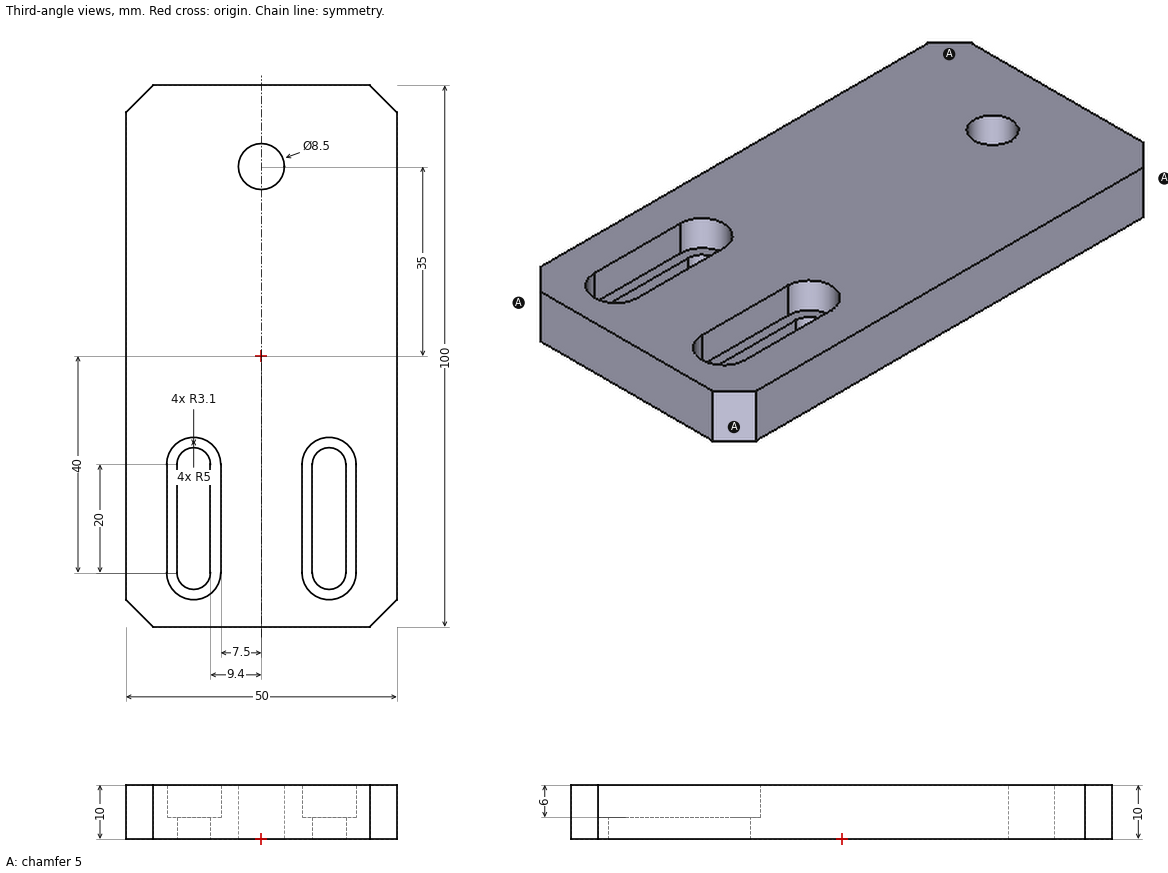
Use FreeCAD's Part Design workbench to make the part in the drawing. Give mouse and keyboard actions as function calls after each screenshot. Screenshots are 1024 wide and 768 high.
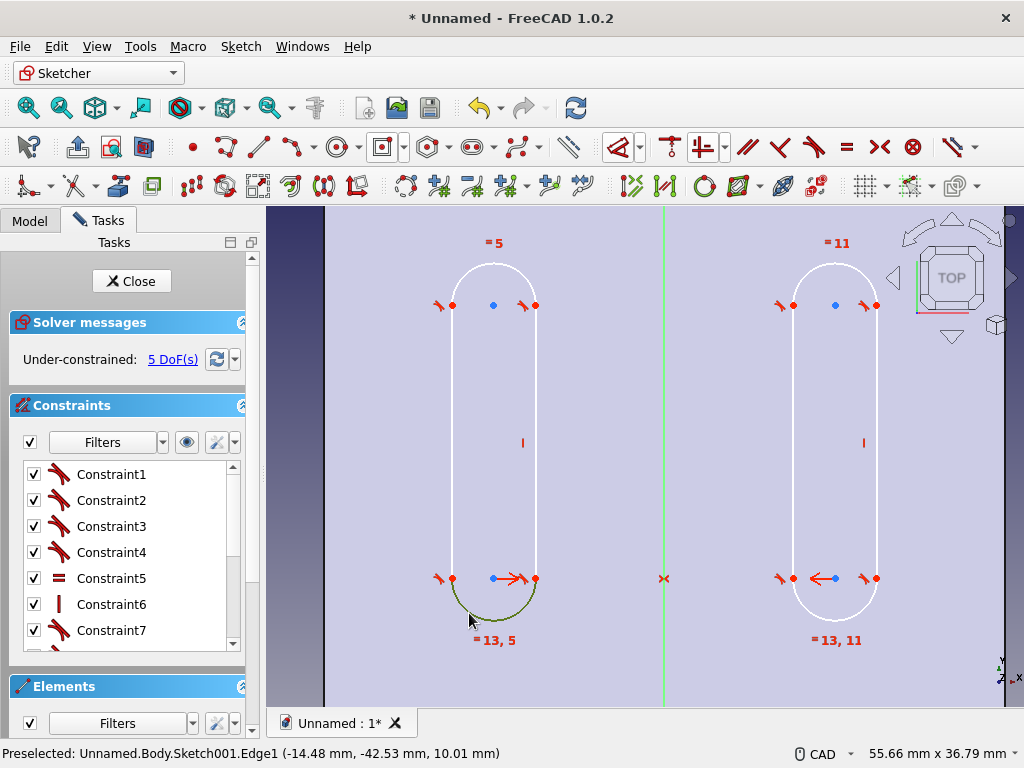
key(k)
key(r)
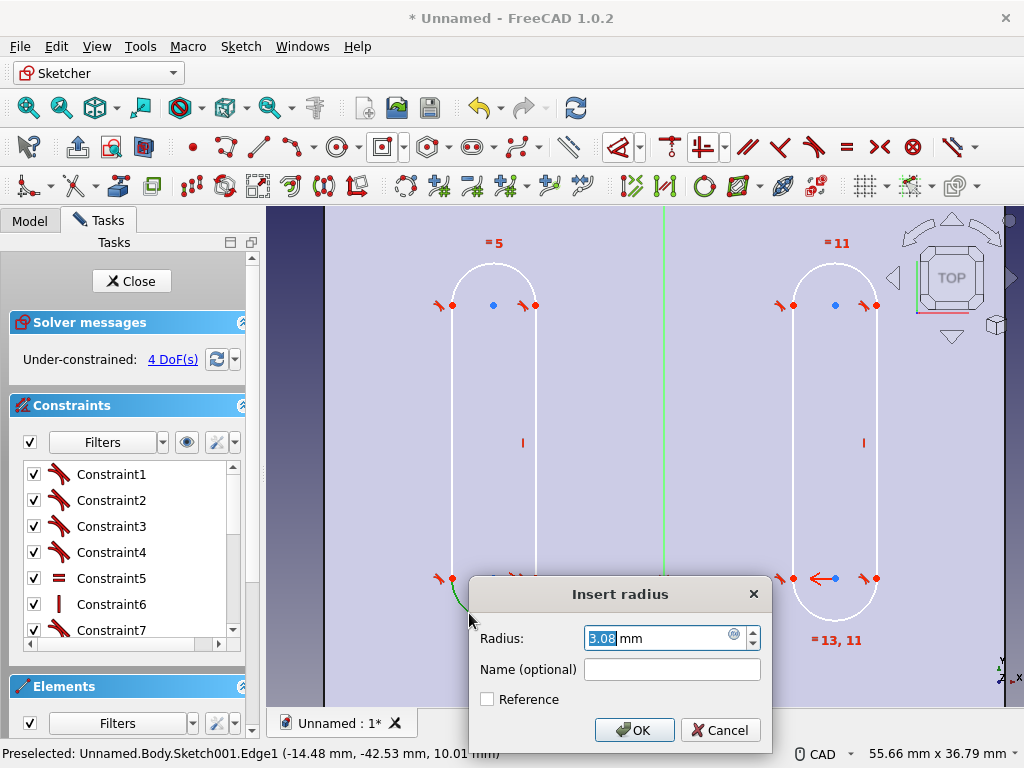
text(3.1)
key(Return)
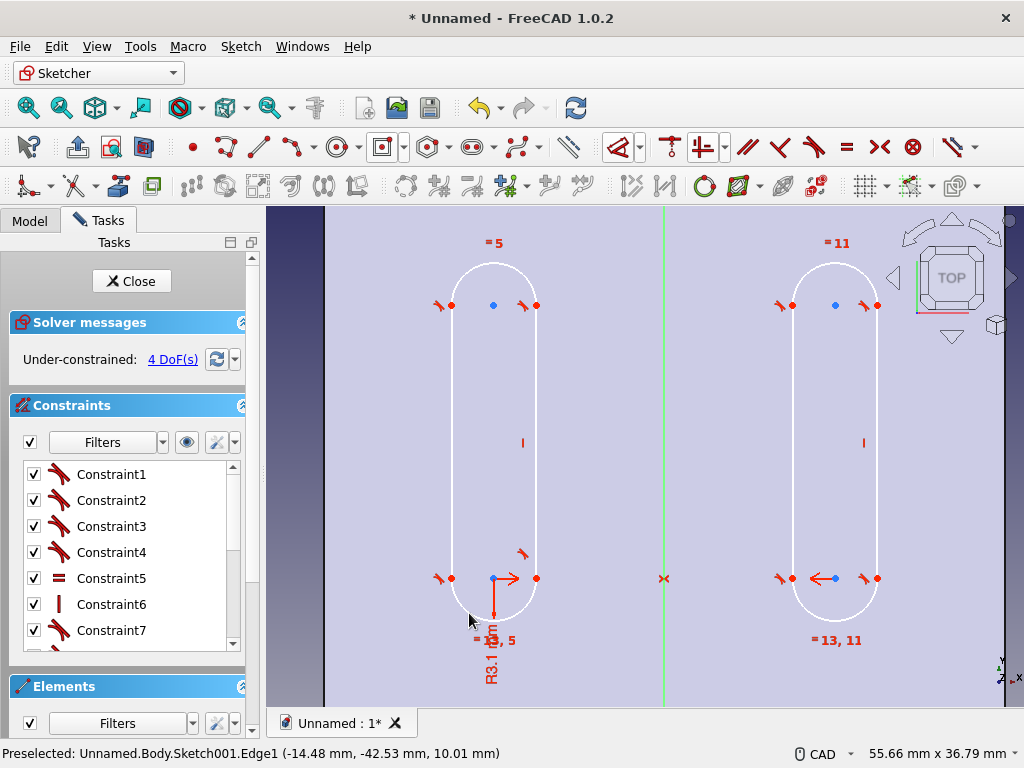
click(452, 497)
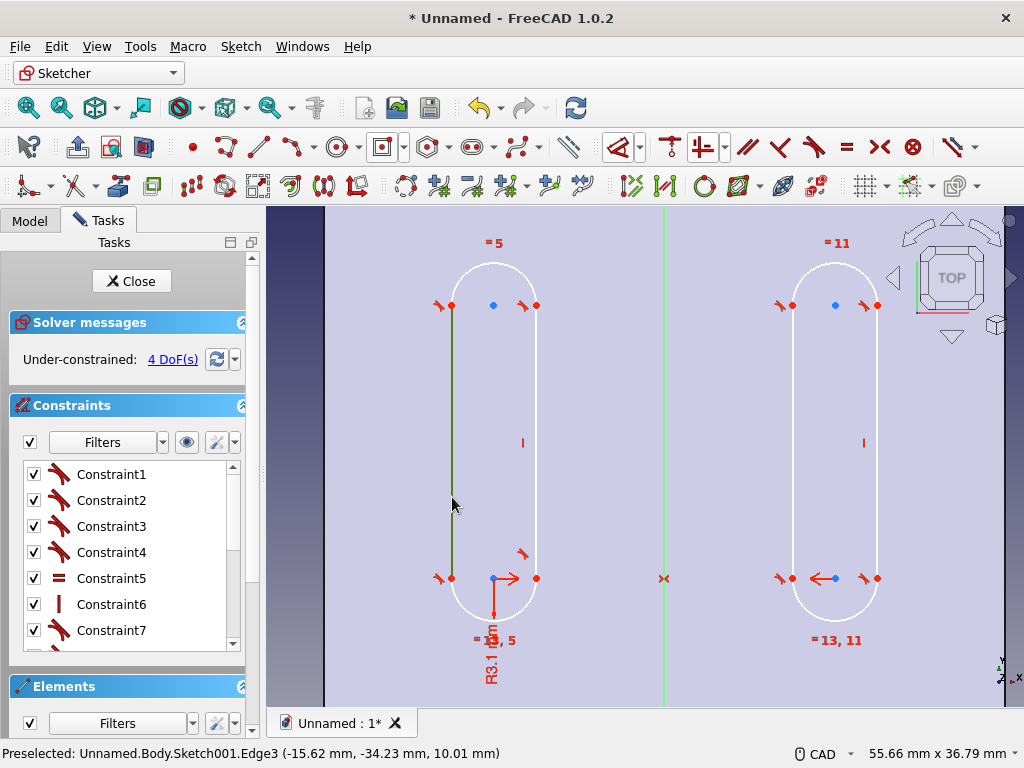
key(i)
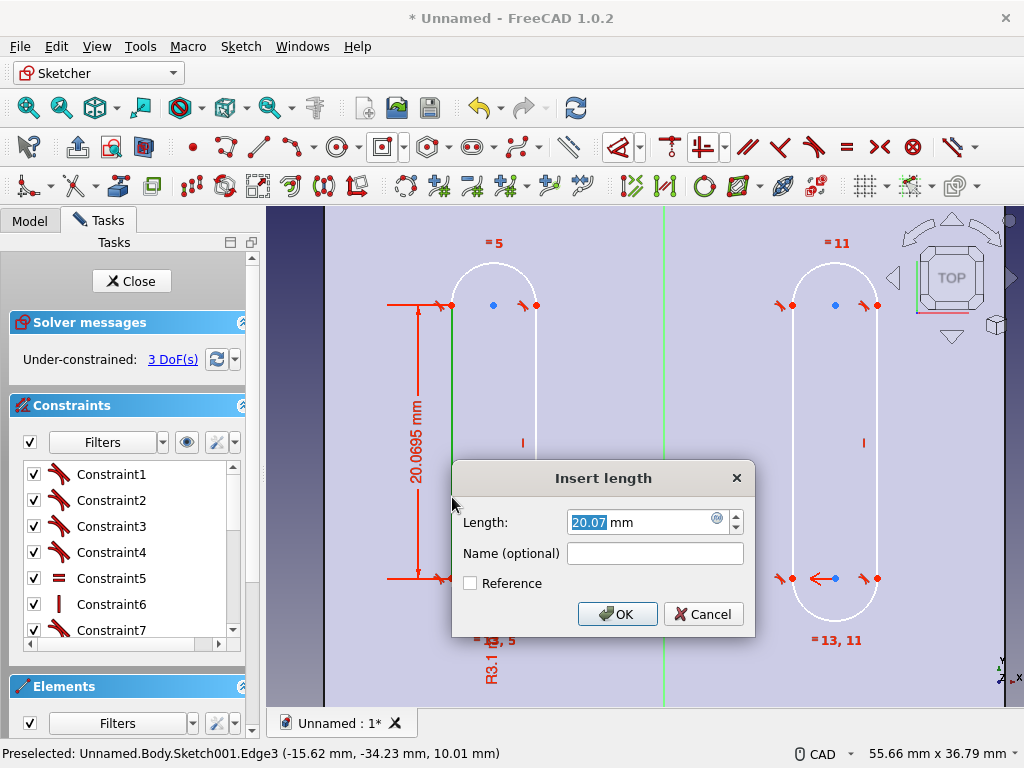
text(20)
key(Return)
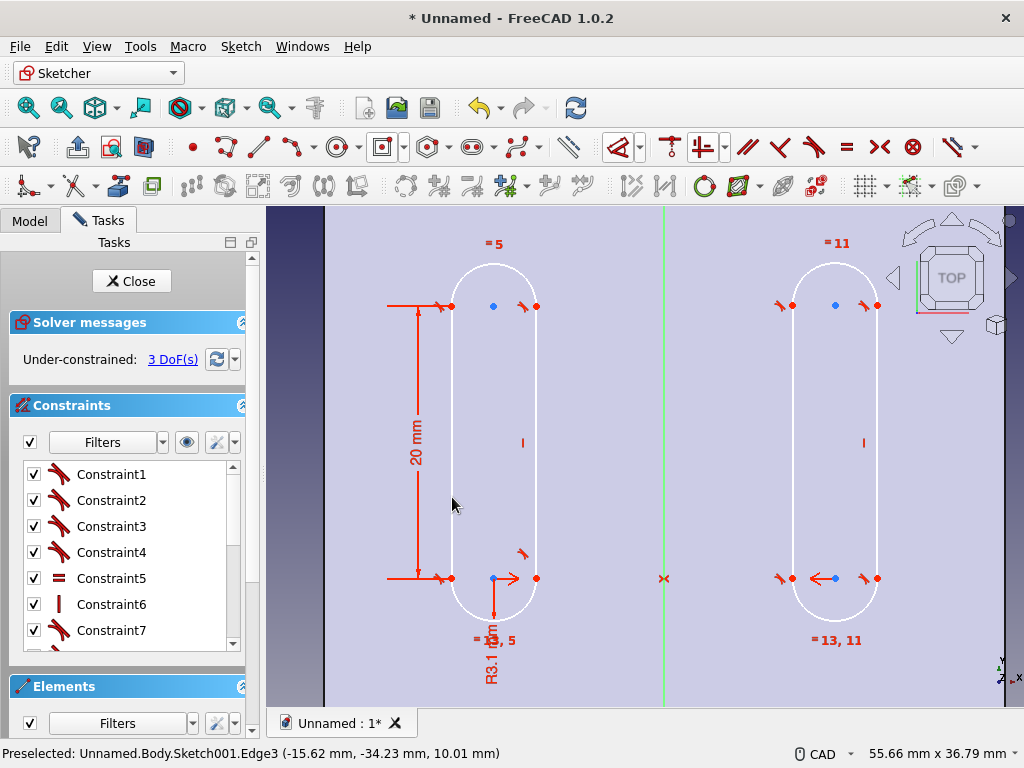
click(793, 497)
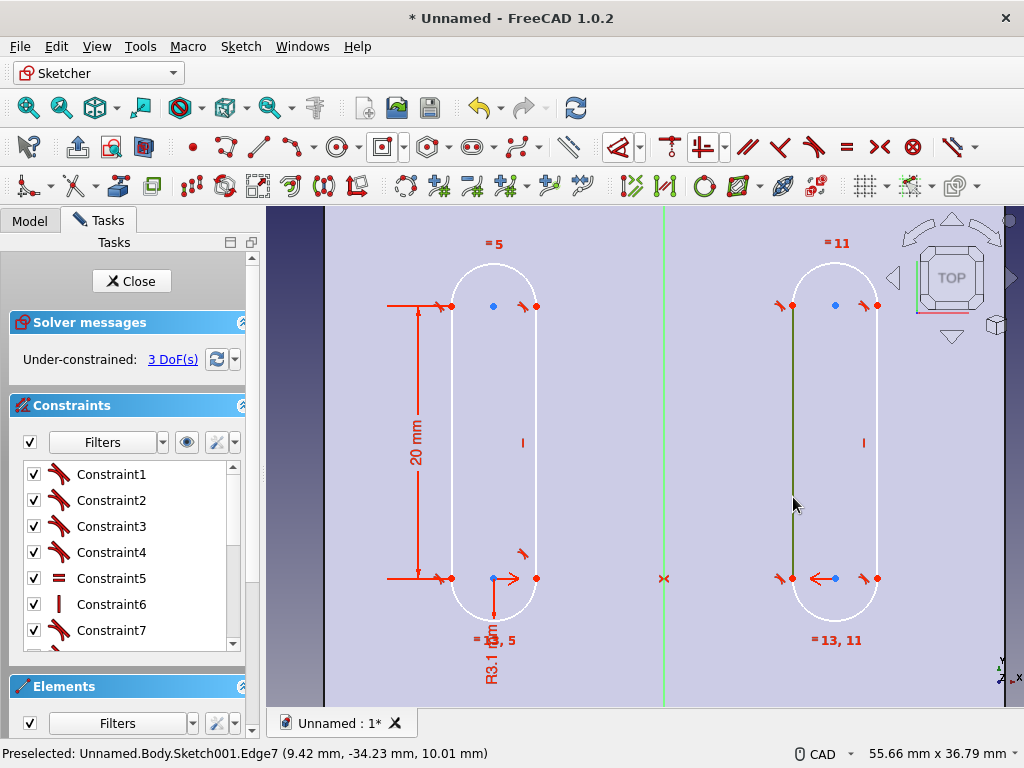
key(i)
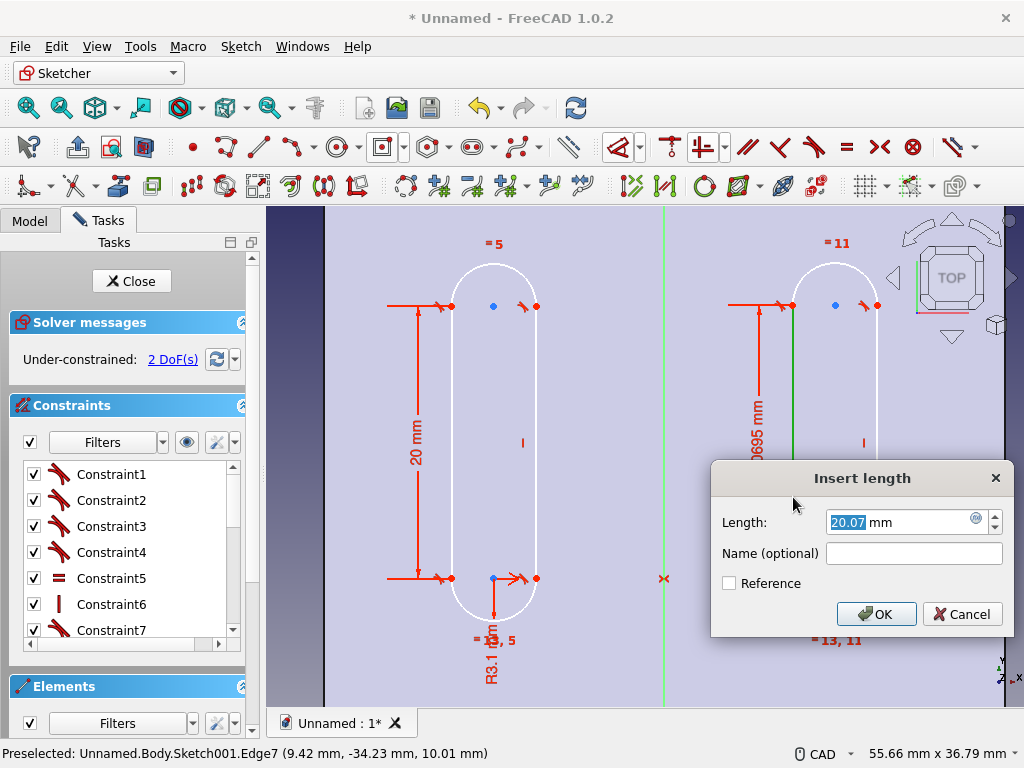
text(20)
key(Return)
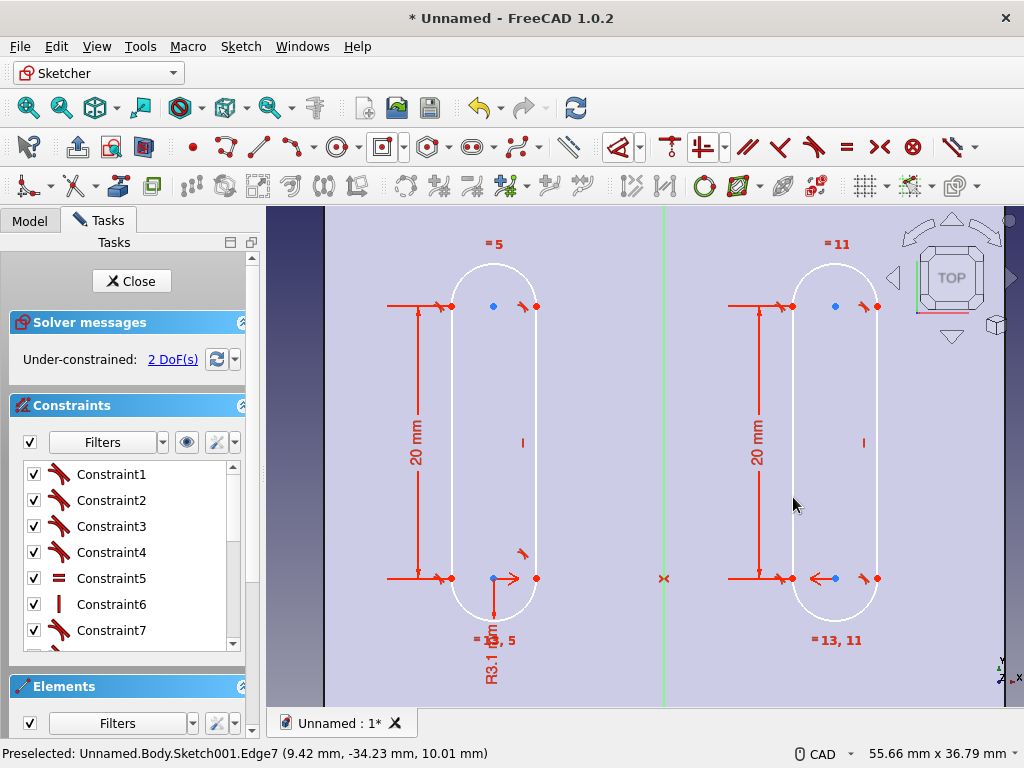
click(452, 579)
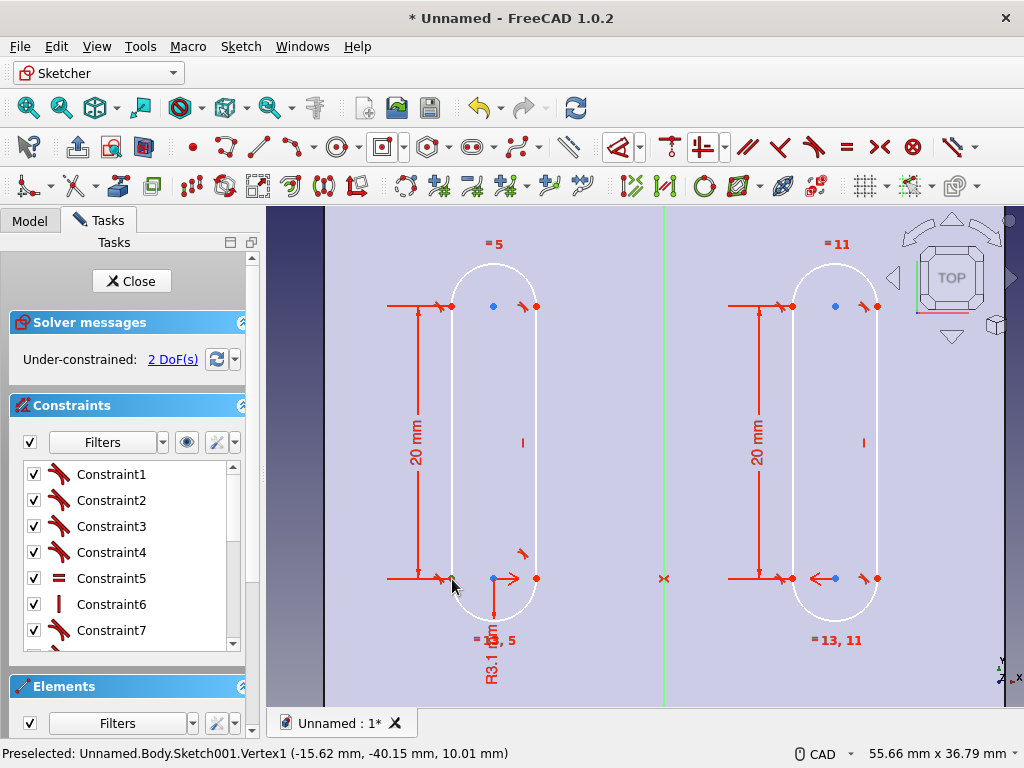
key(i)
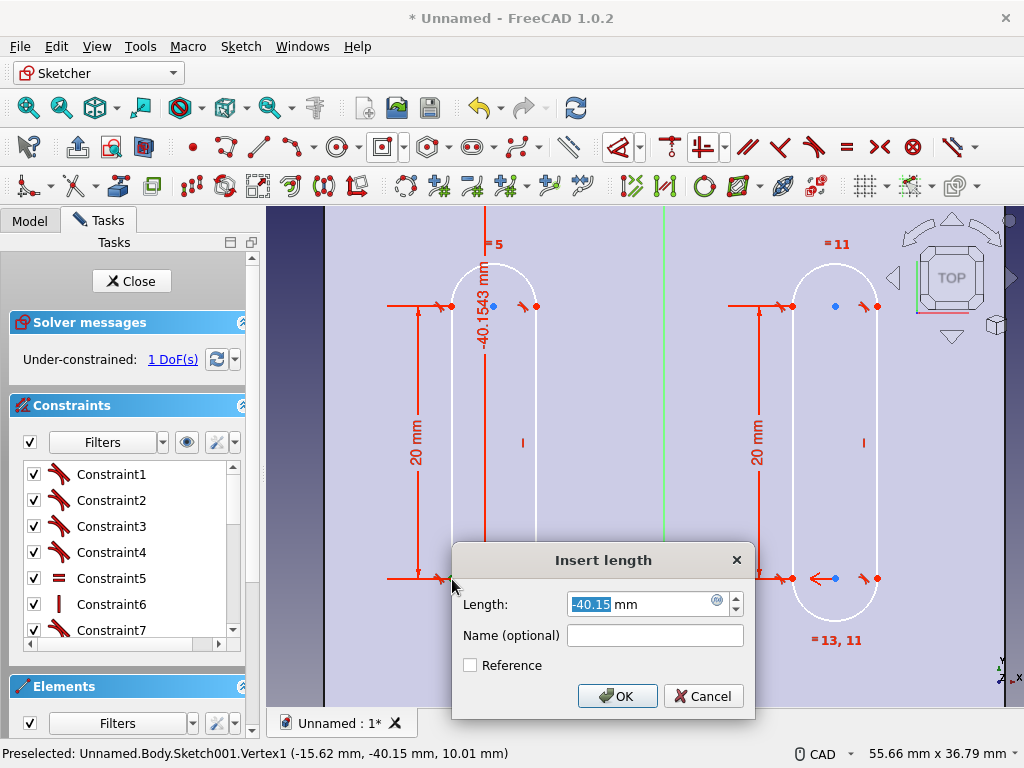
text(-40)
key(Return)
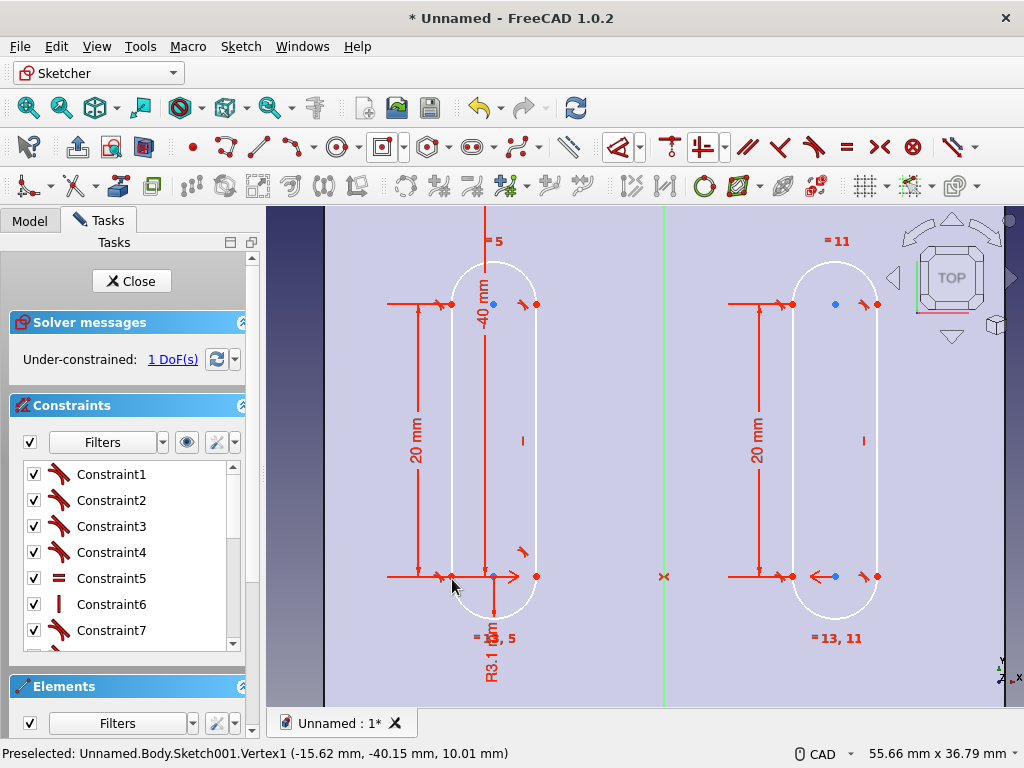
click(536, 577)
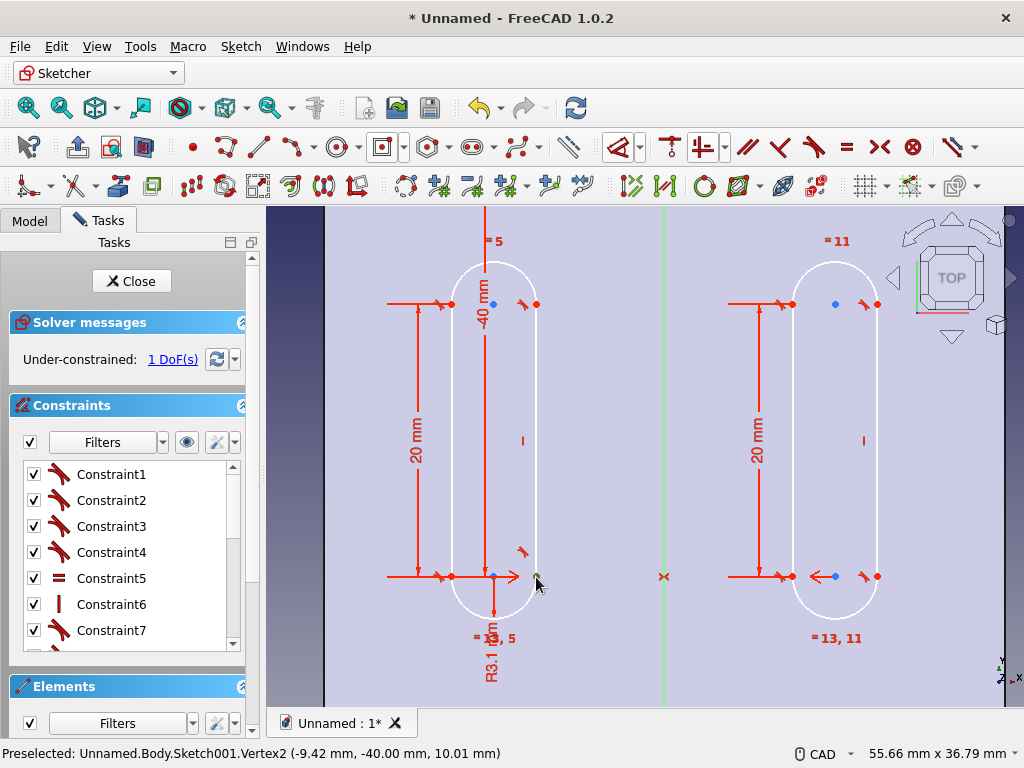
key(l)